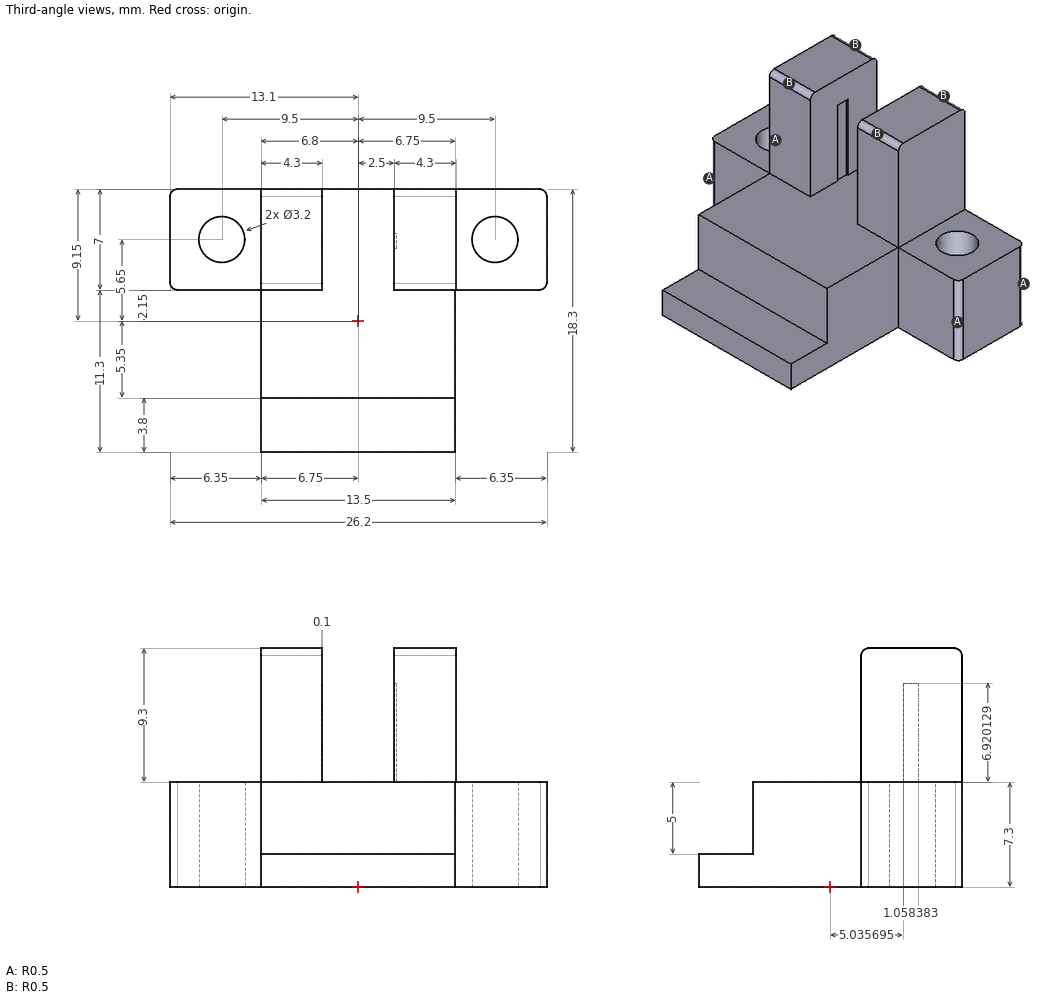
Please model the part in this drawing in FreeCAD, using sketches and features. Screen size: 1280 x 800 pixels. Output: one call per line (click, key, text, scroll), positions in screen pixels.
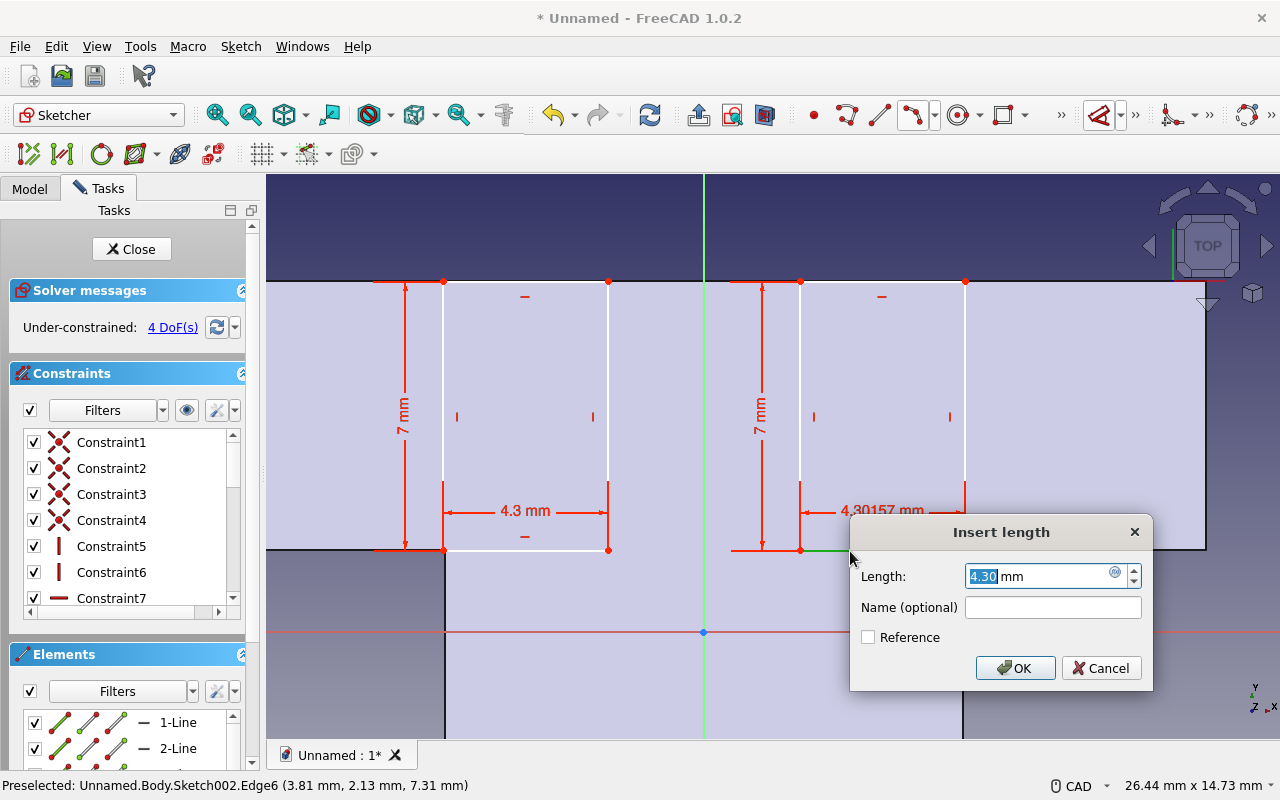
text(4.3)
key(Return)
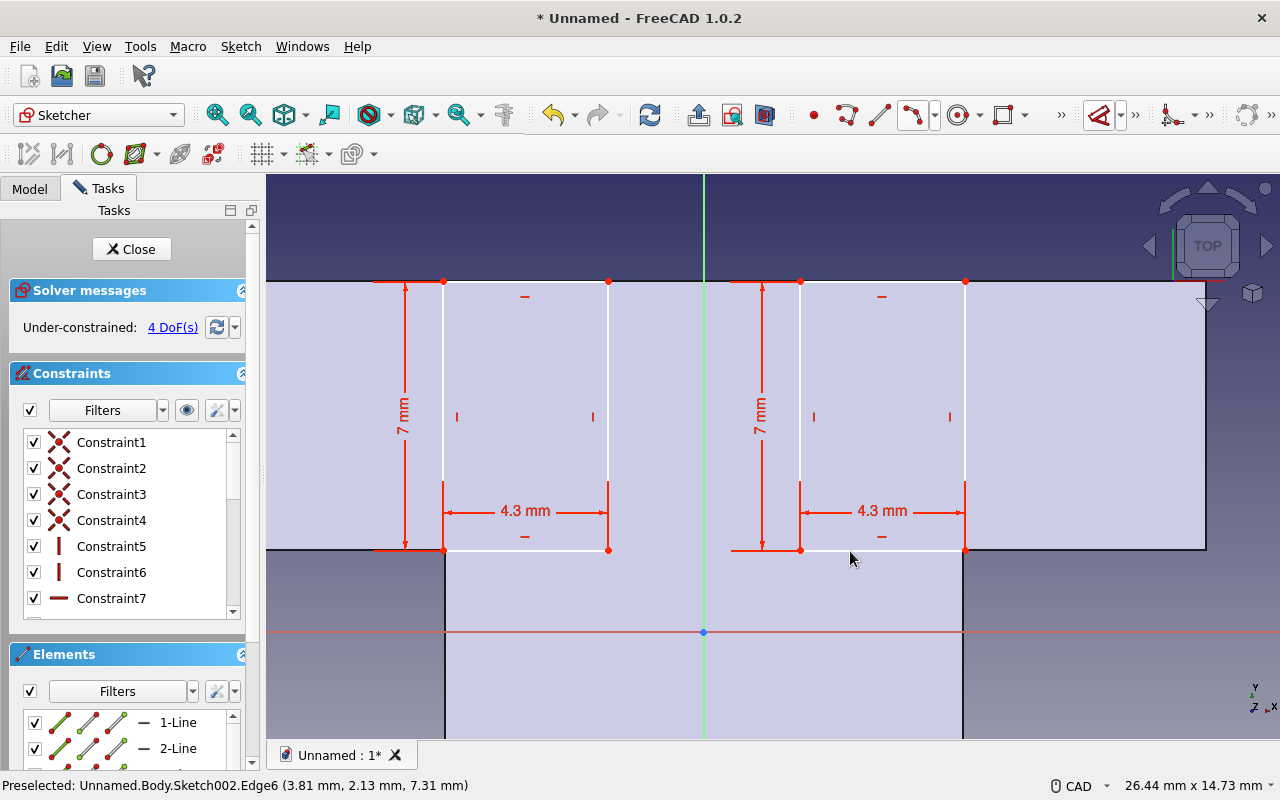
click(443, 282)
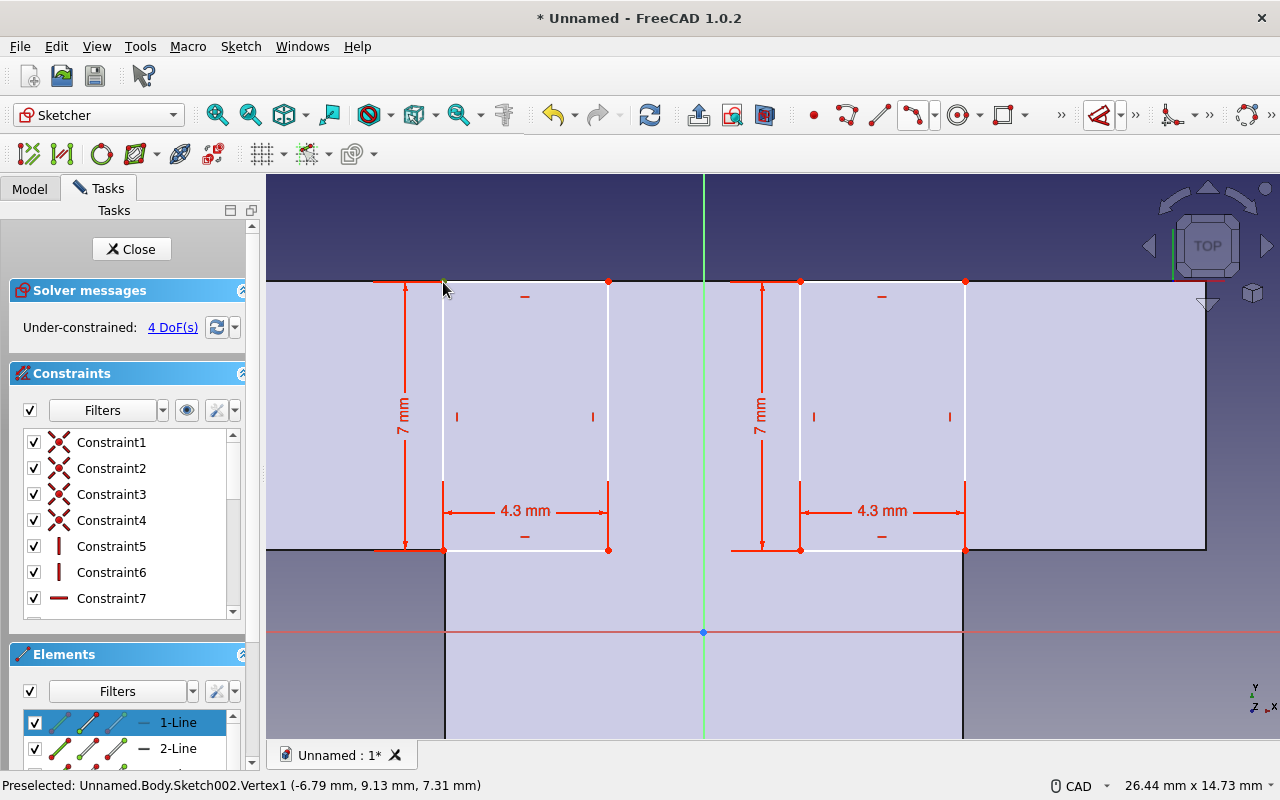
key(l)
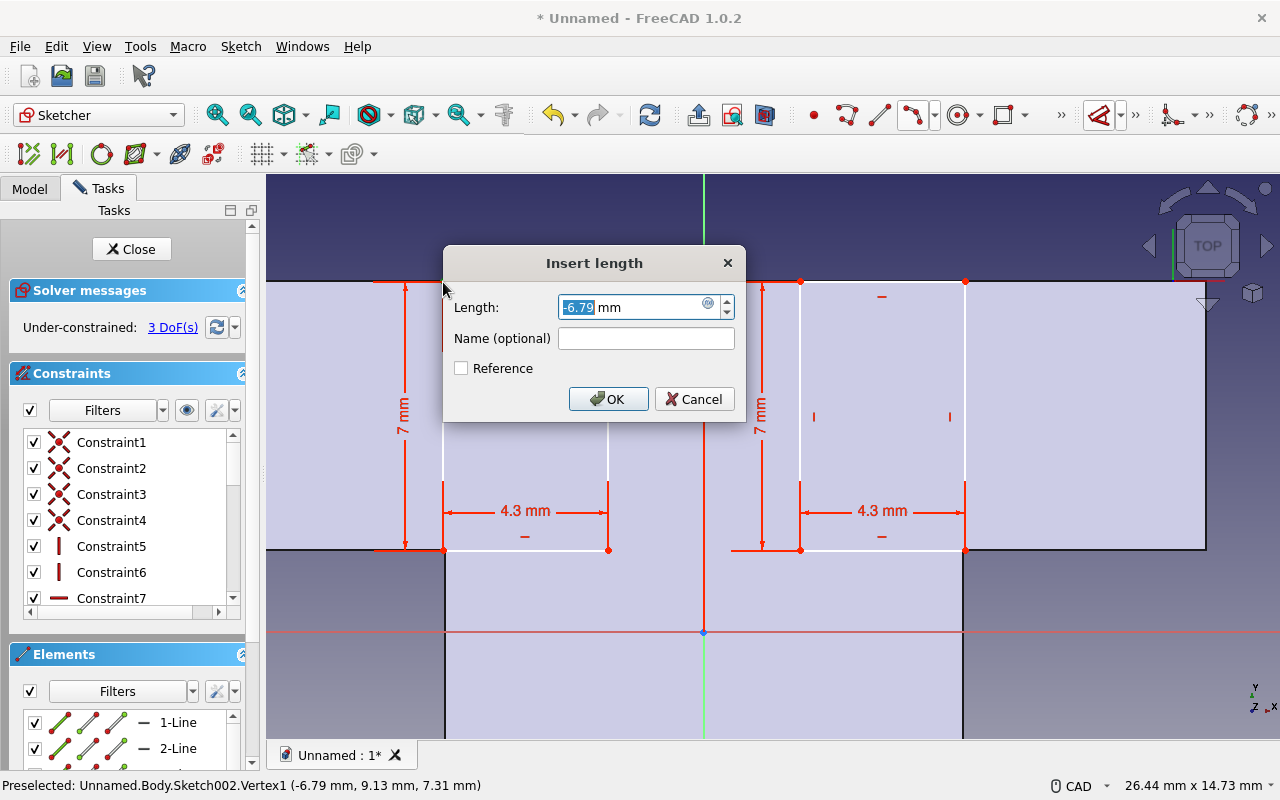
text(-6.8)
key(Return)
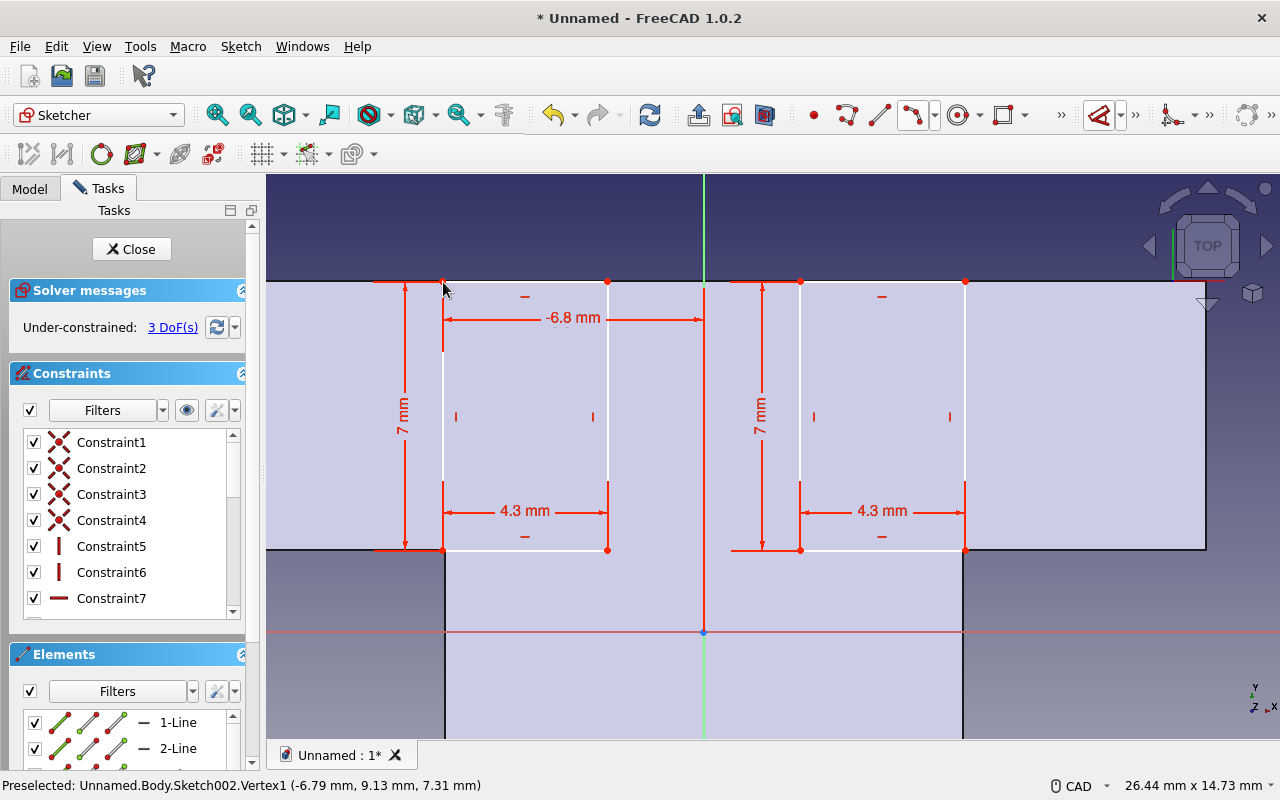
click(800, 282)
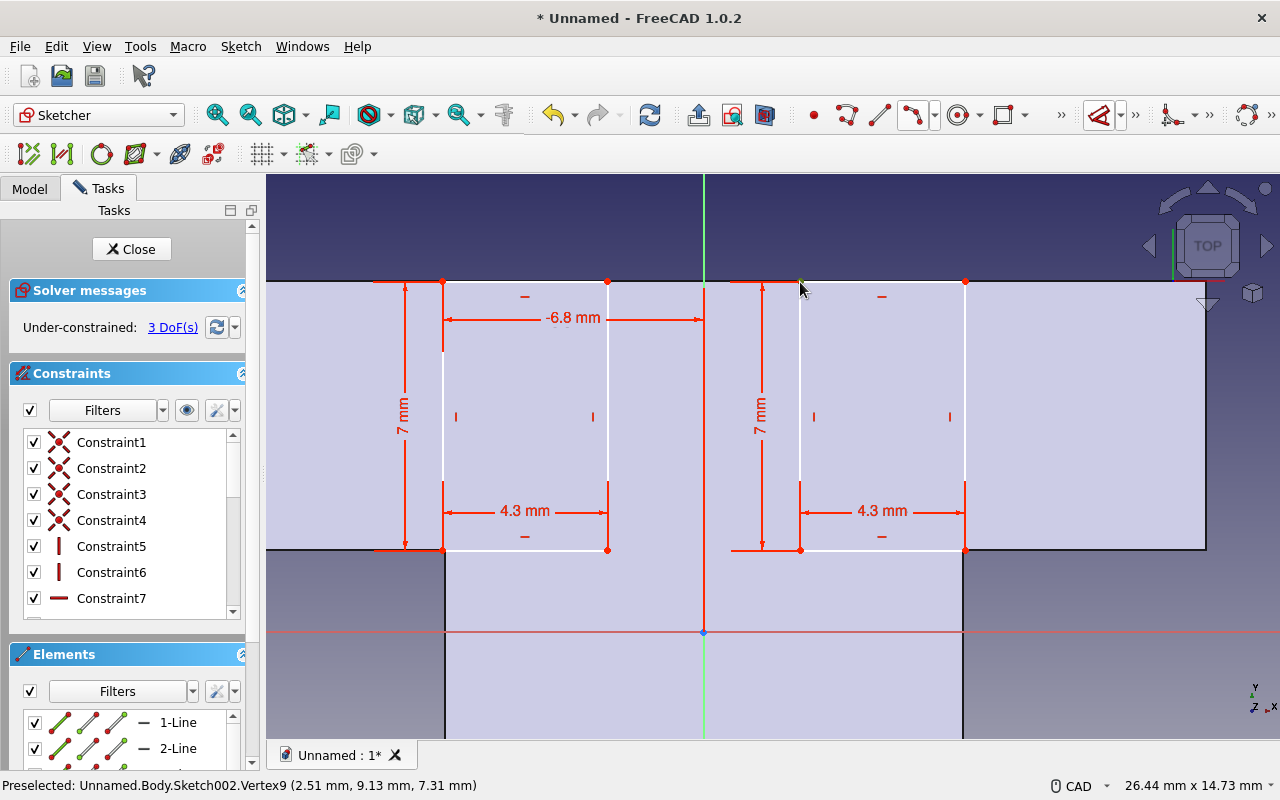
key(l)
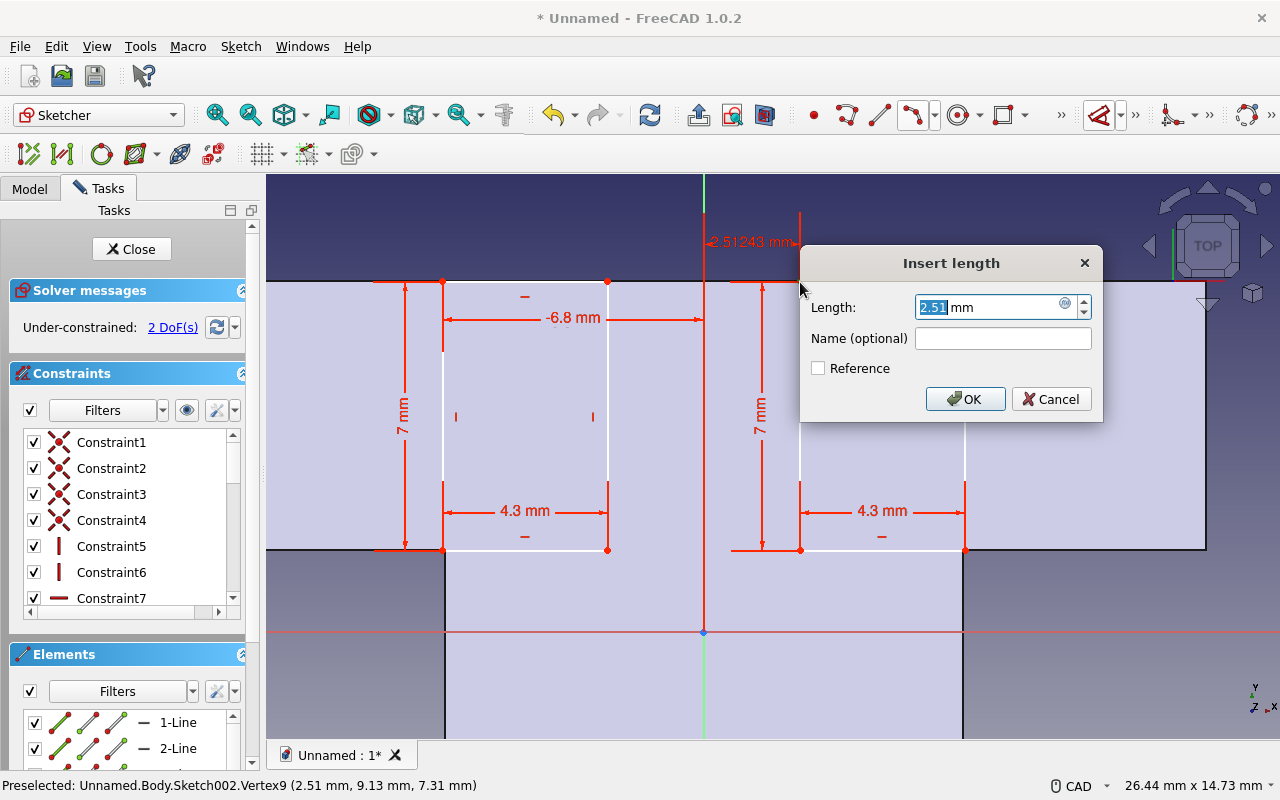
text(2.5)
key(Return)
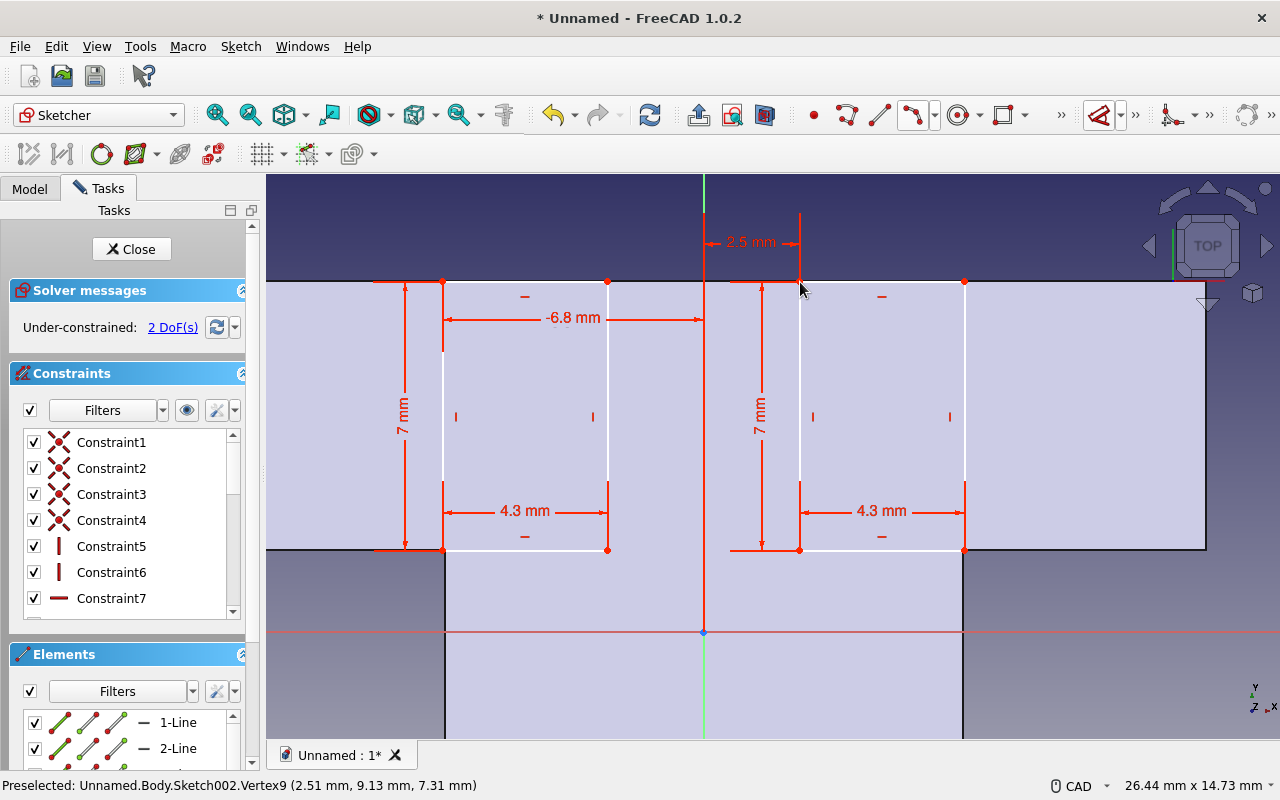
click(443, 282)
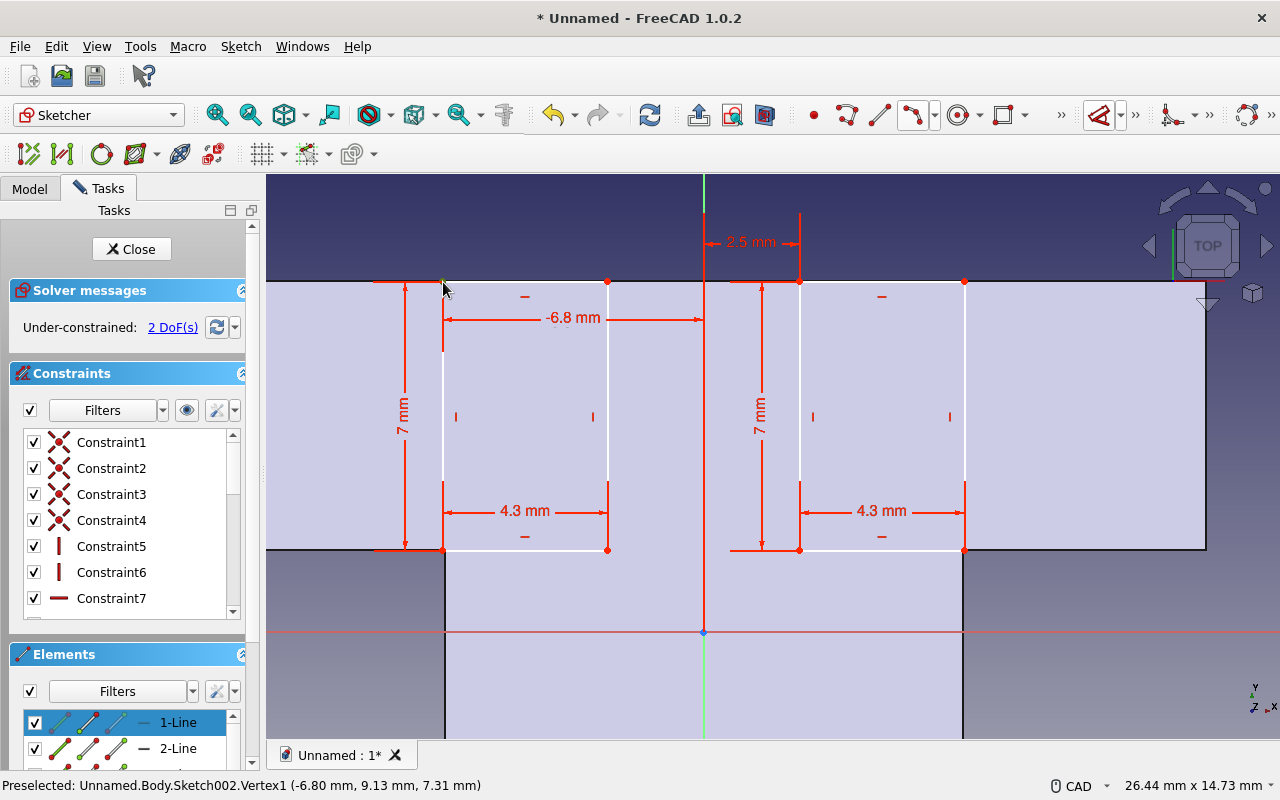
key(i)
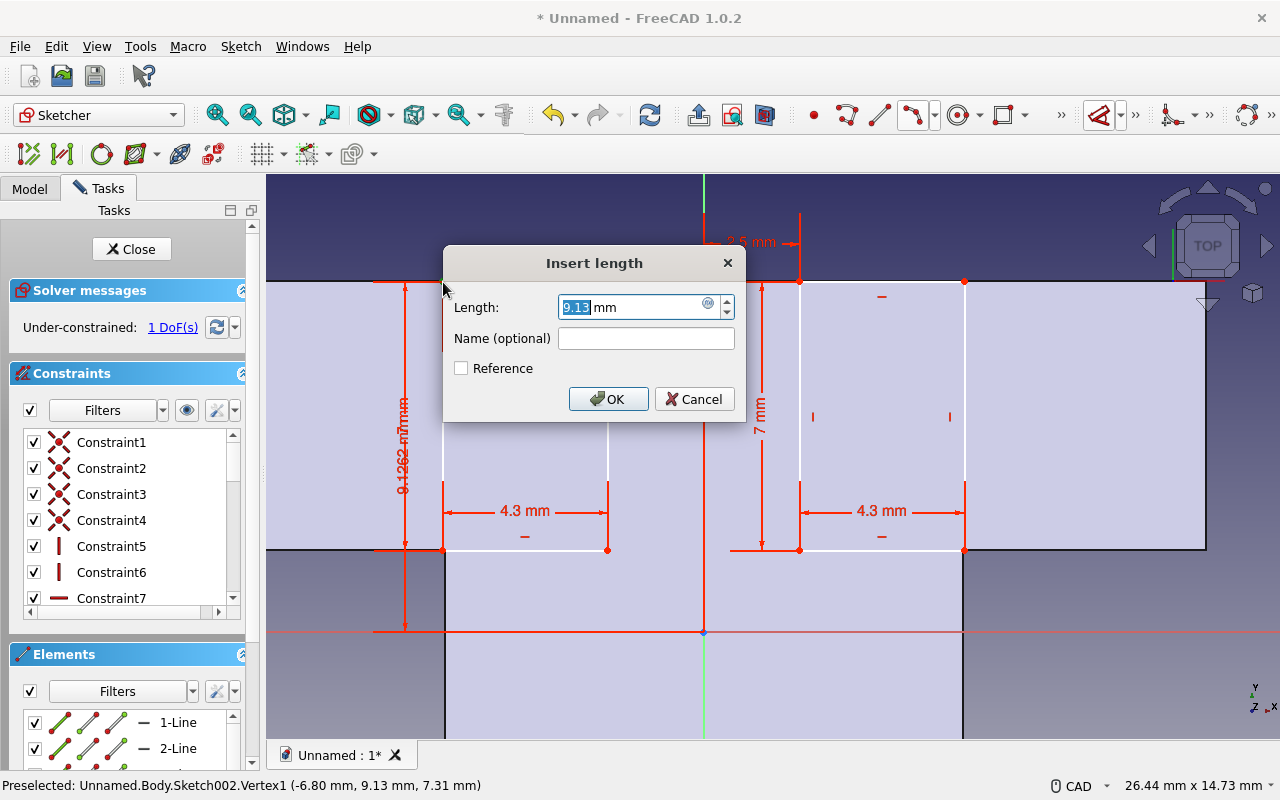
text(9.15)
key(Return)